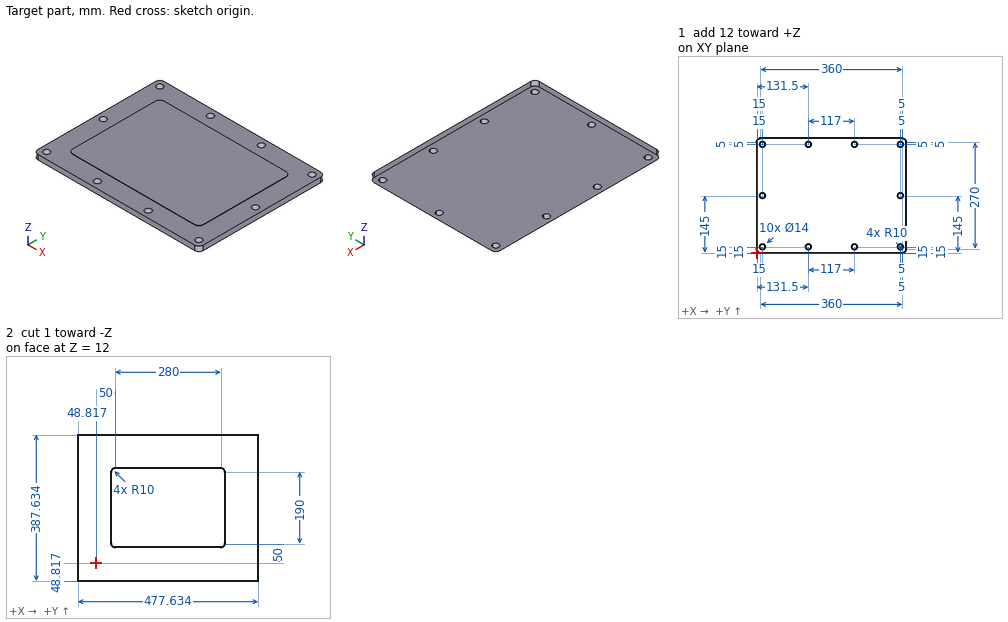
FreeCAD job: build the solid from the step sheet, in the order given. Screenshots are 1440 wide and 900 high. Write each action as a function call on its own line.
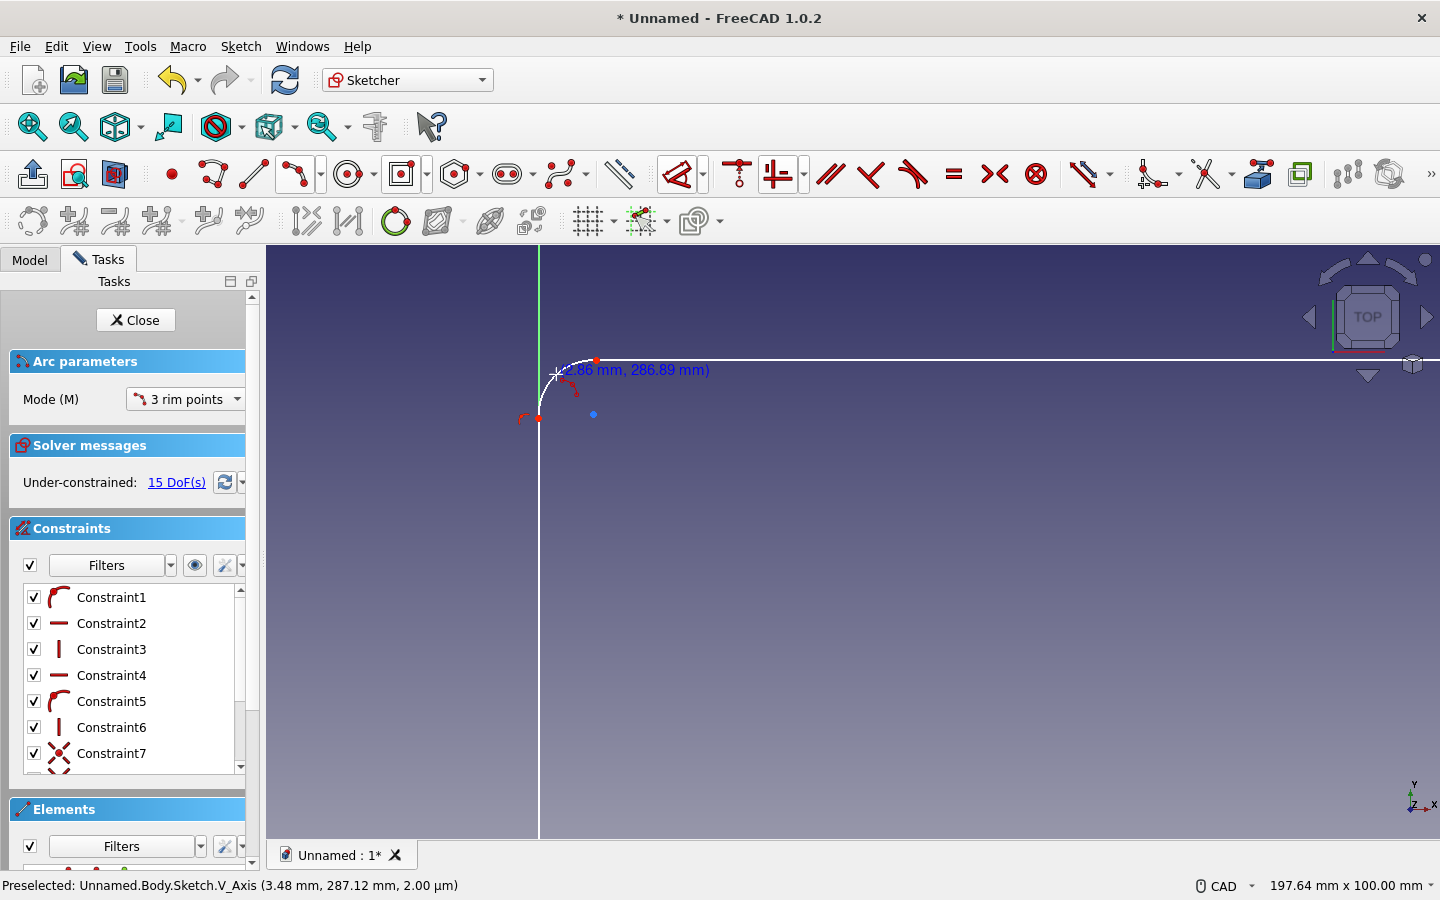
scroll(561, 371, down, 8)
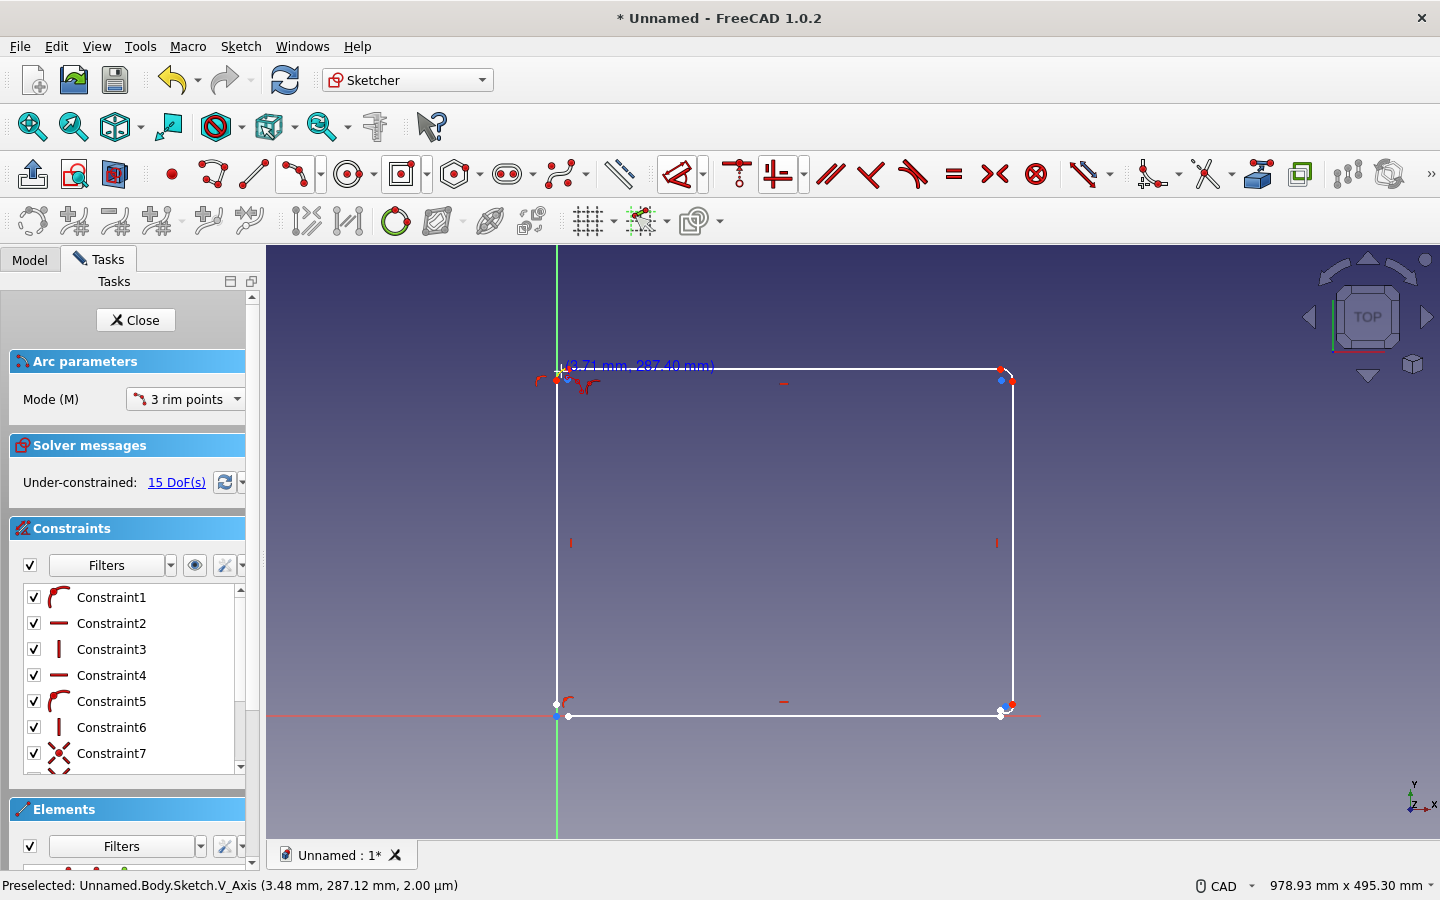
scroll(557, 704, up, 2)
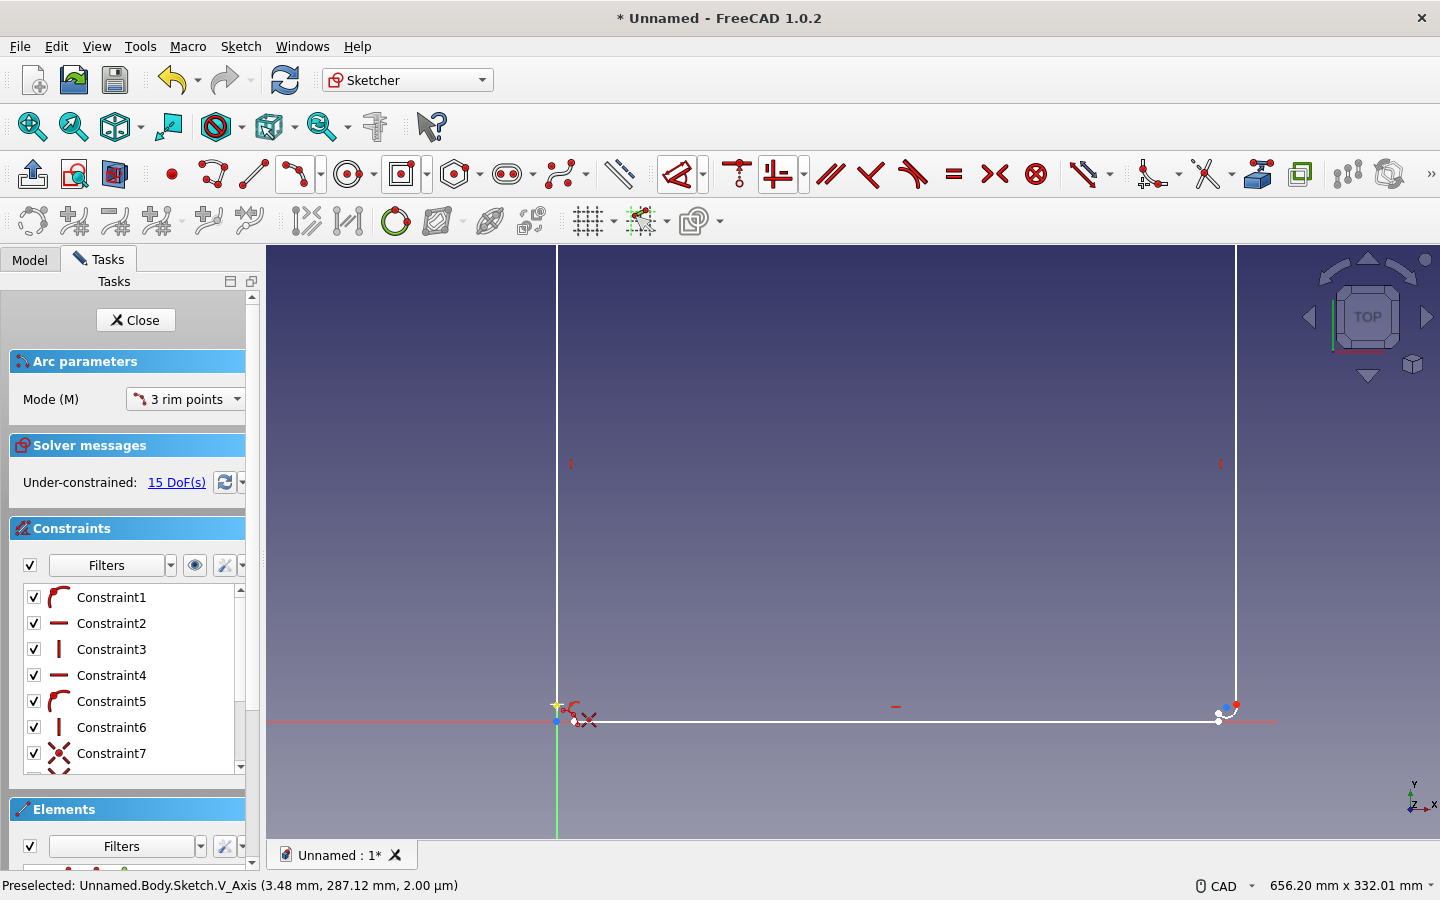
click(557, 705)
click(574, 722)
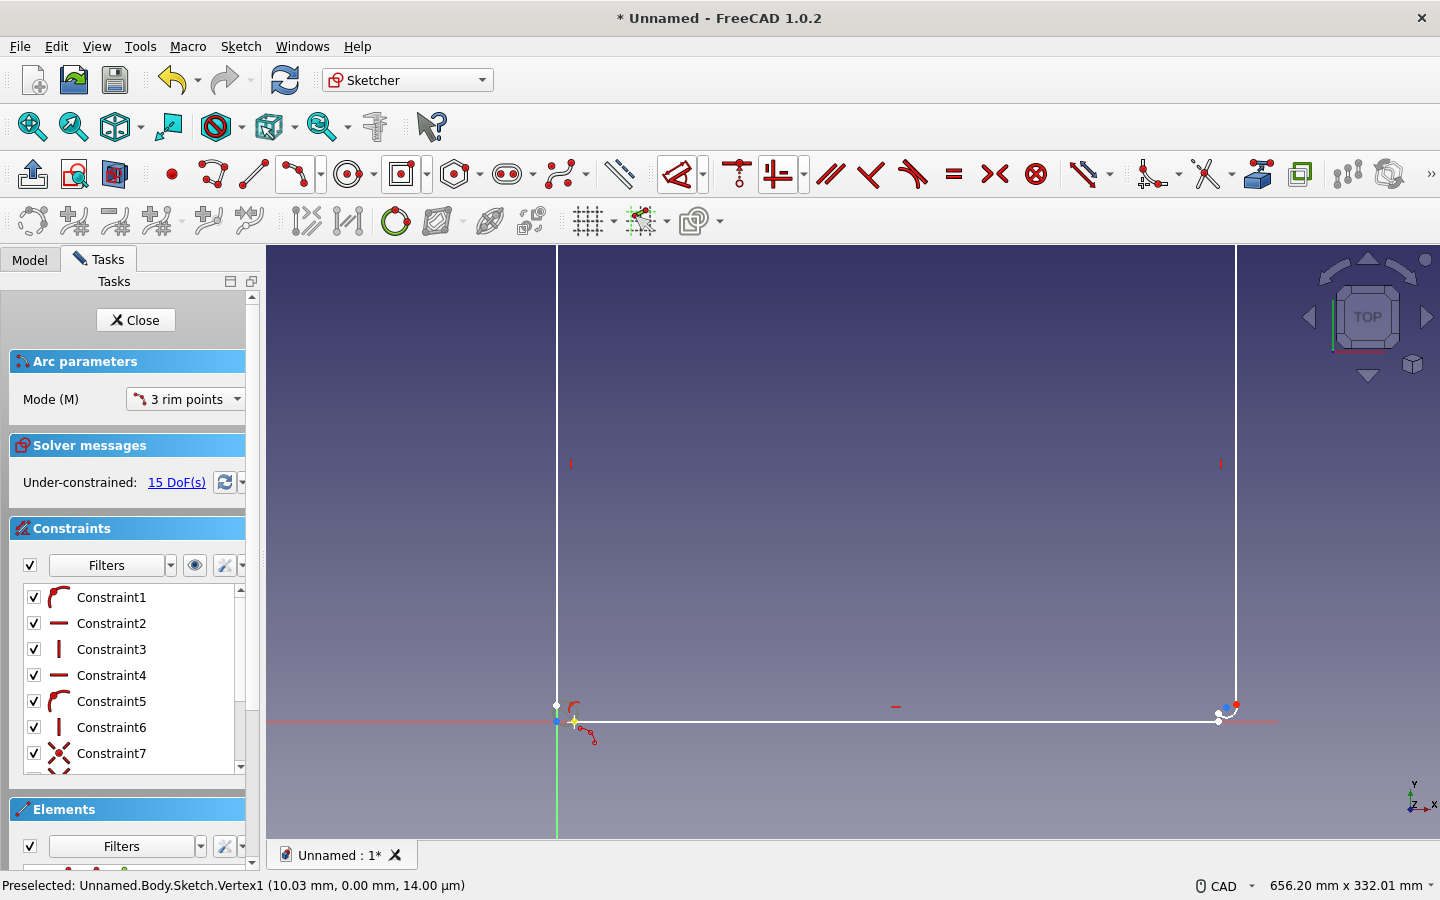
scroll(562, 716, up, 6)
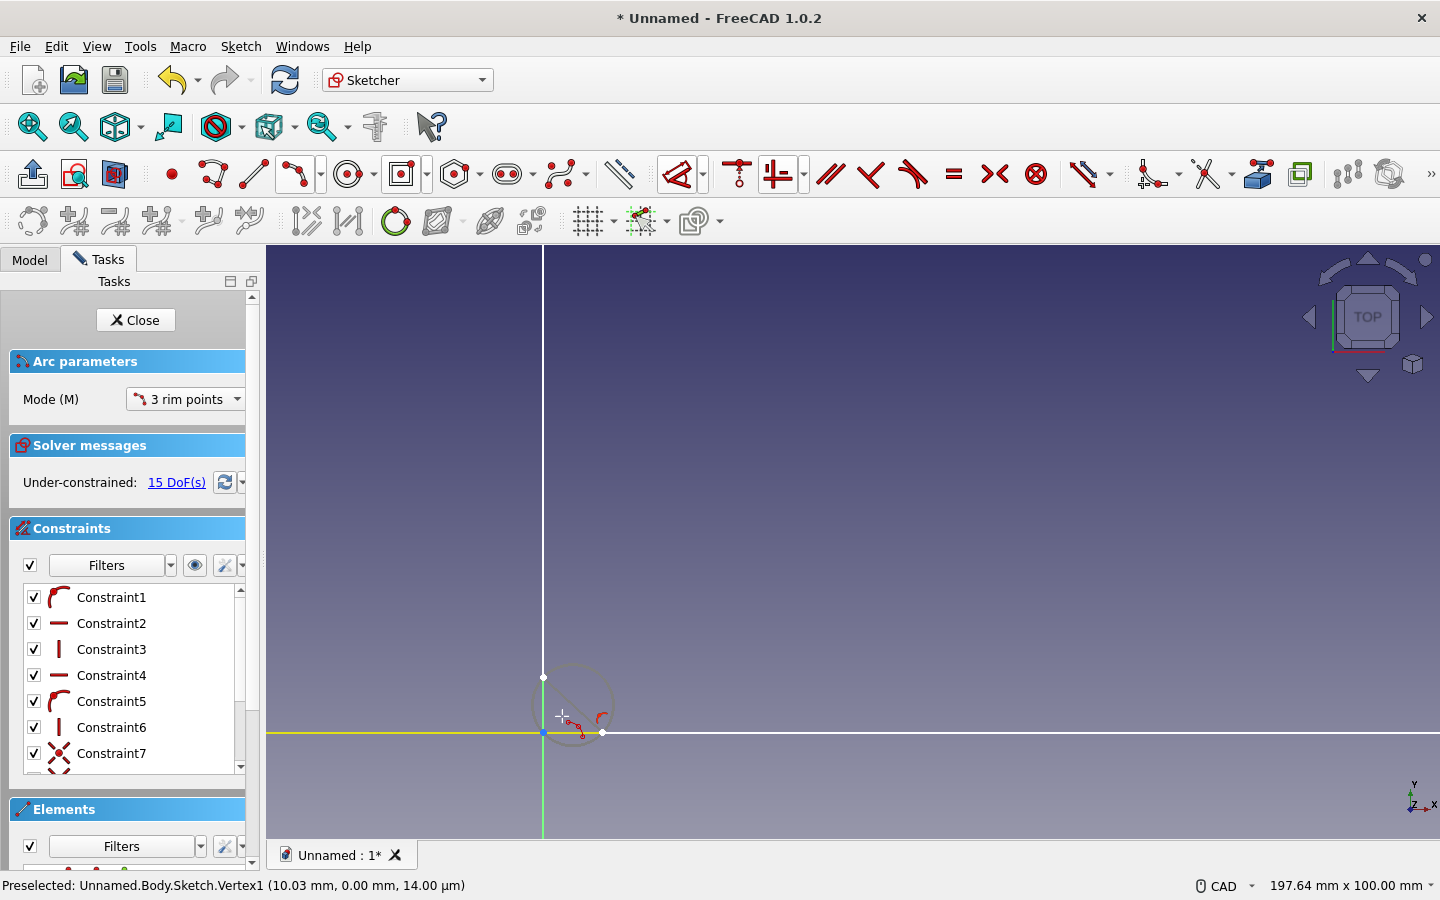
click(561, 715)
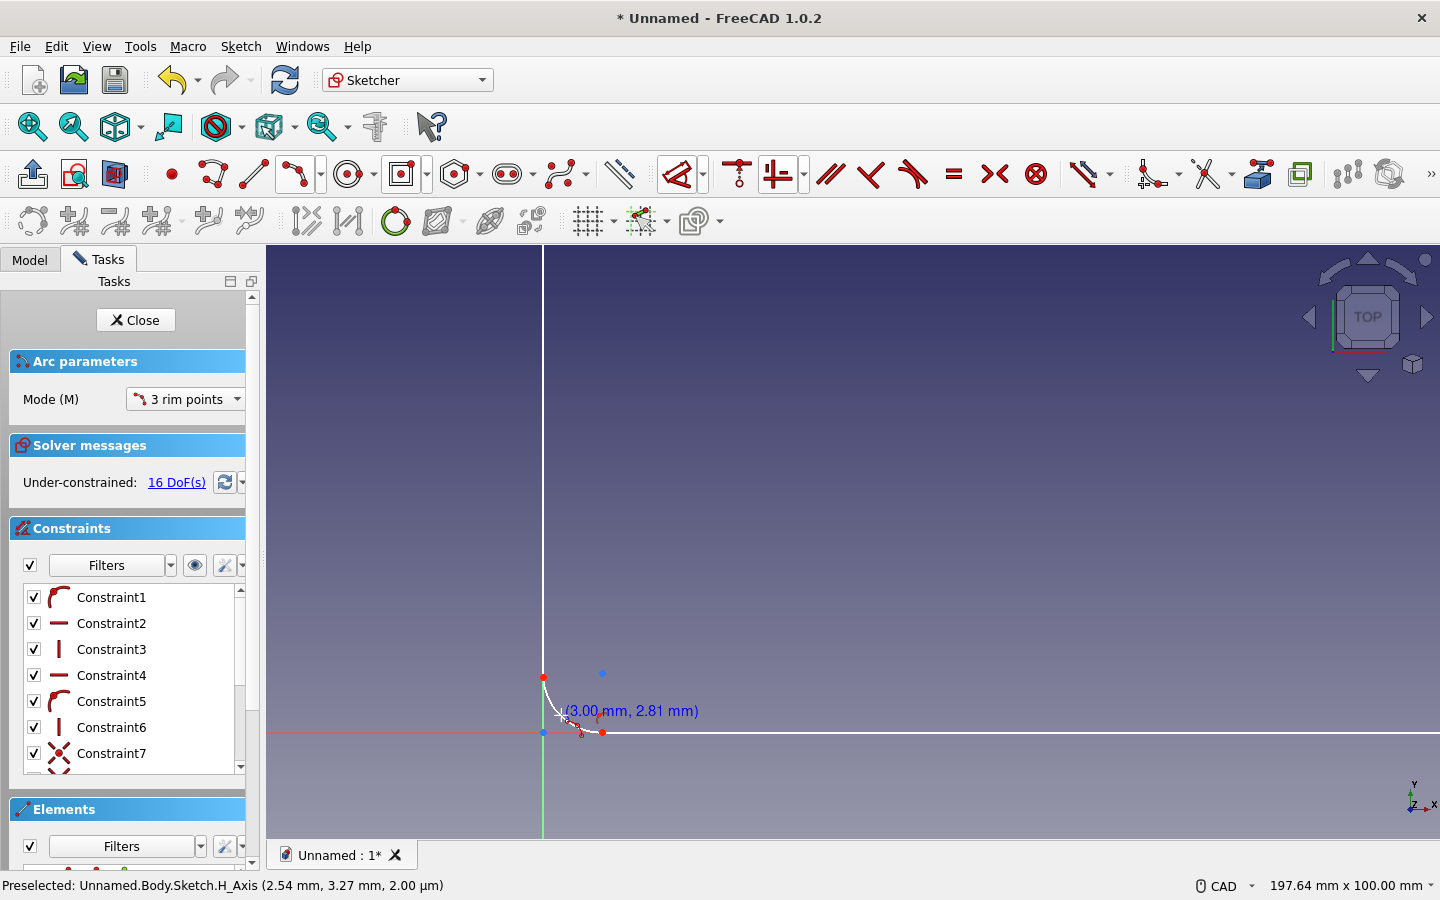
click(348, 174)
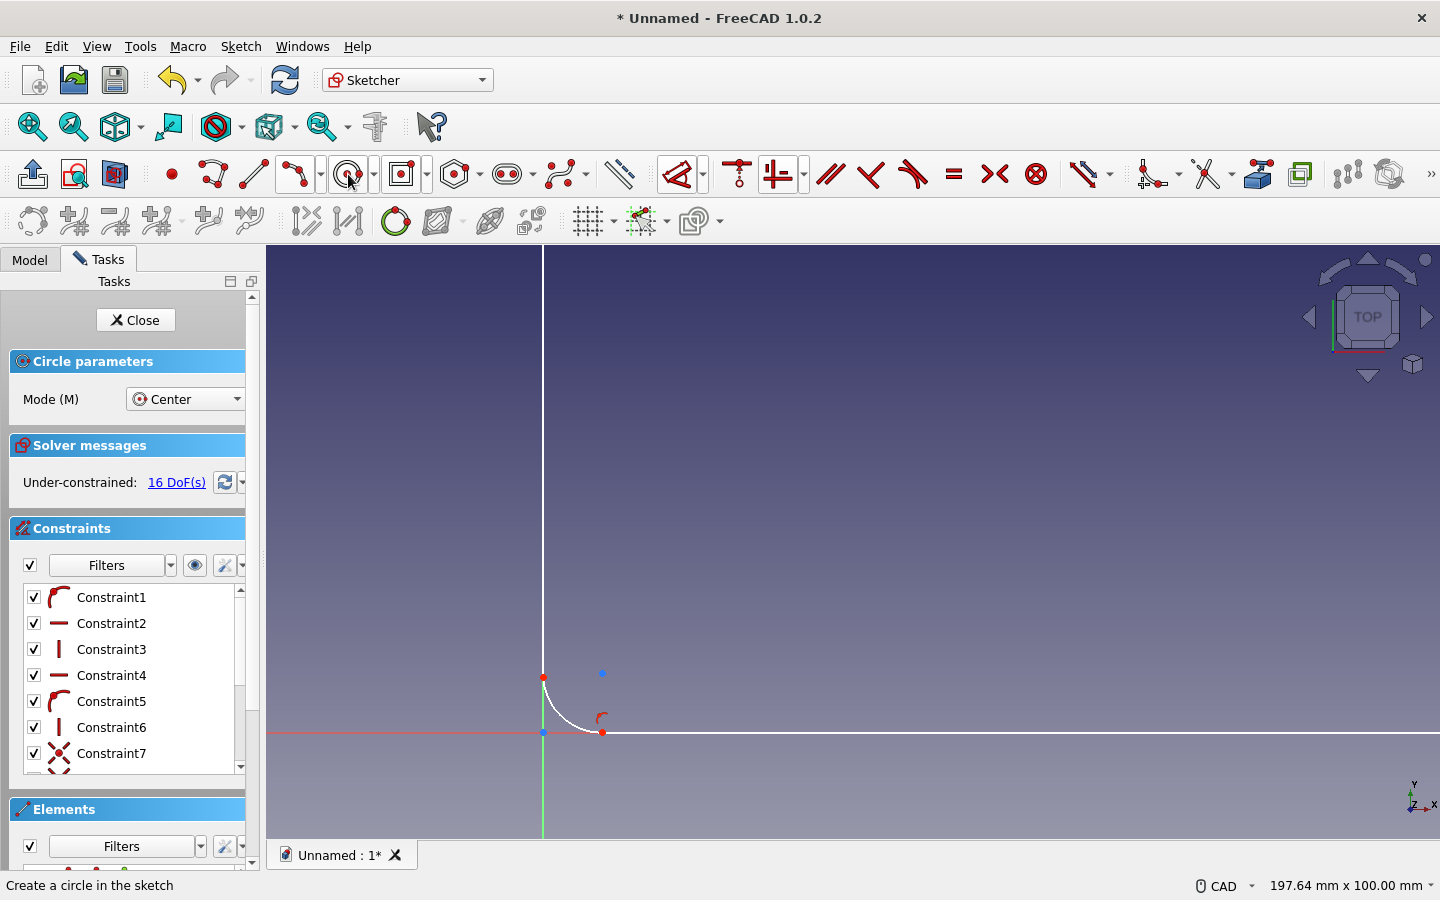
click(632, 644)
click(662, 614)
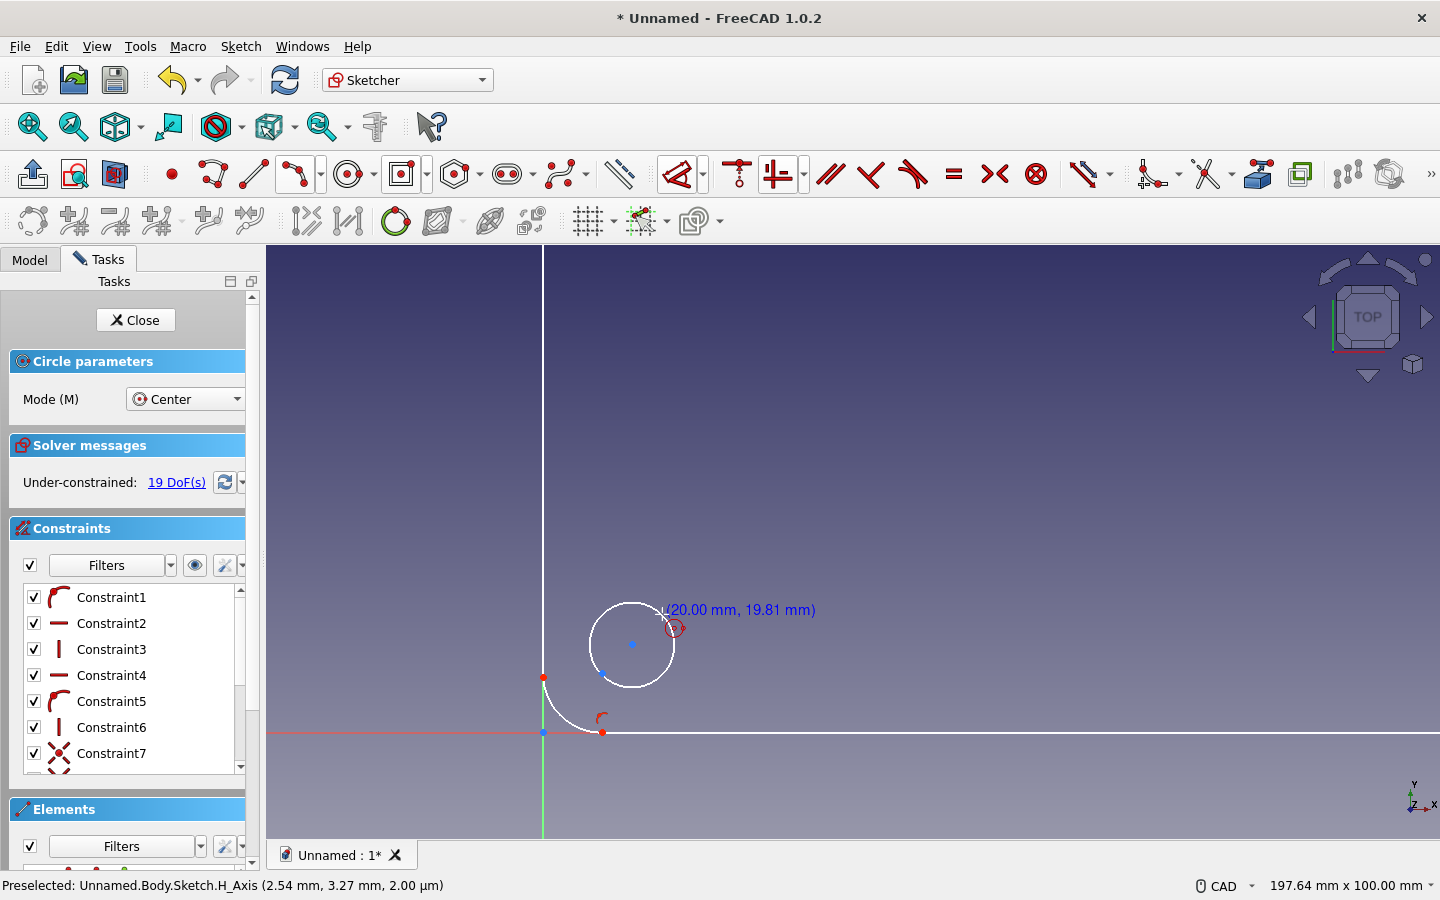
scroll(560, 712, down, 8)